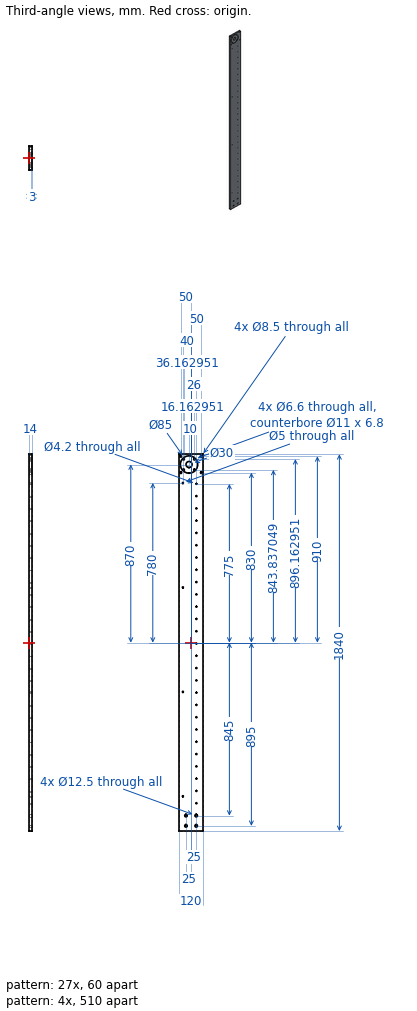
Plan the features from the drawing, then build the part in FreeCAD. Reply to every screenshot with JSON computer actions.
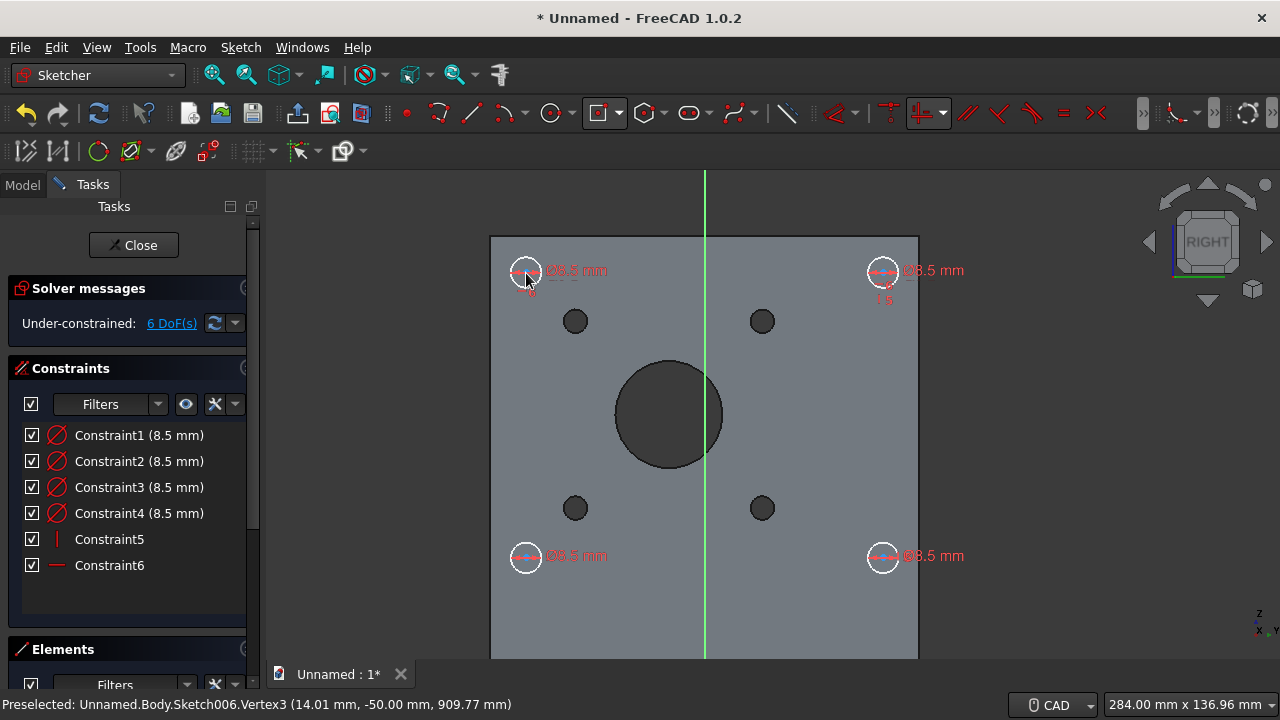
{"action": "left_click", "coordinate": [526, 273]}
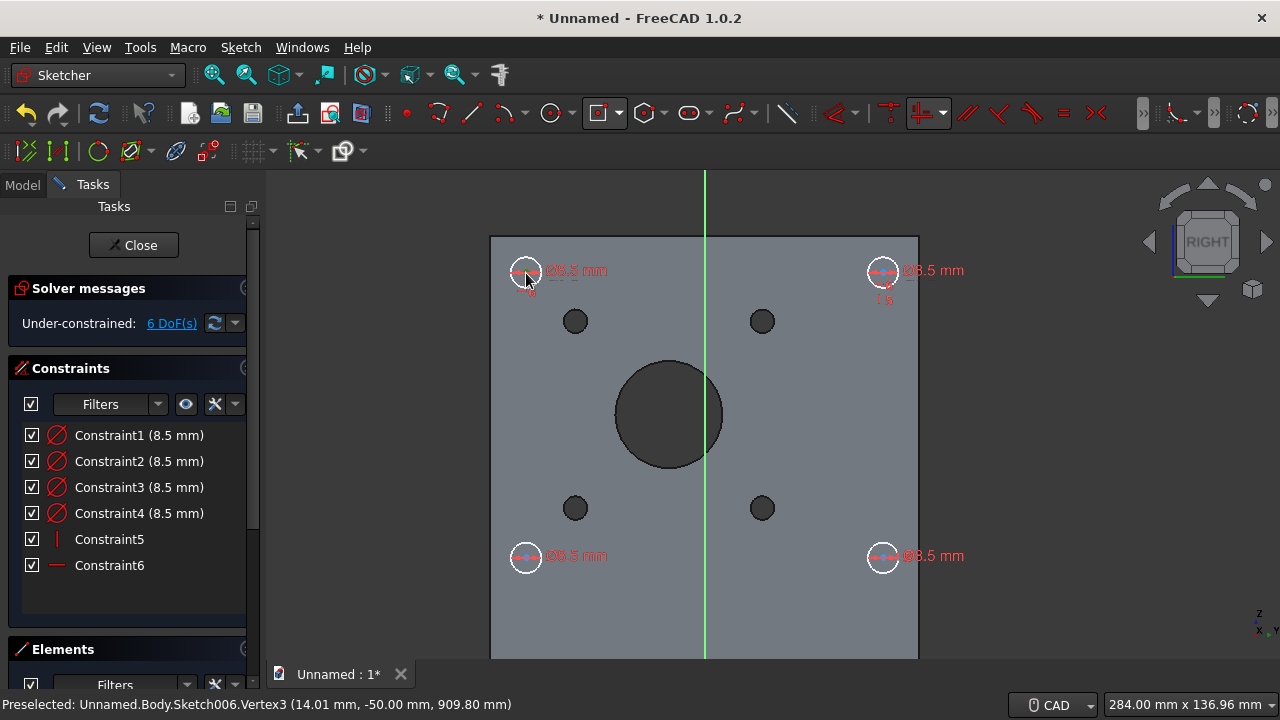
{"action": "left_click", "coordinate": [526, 558]}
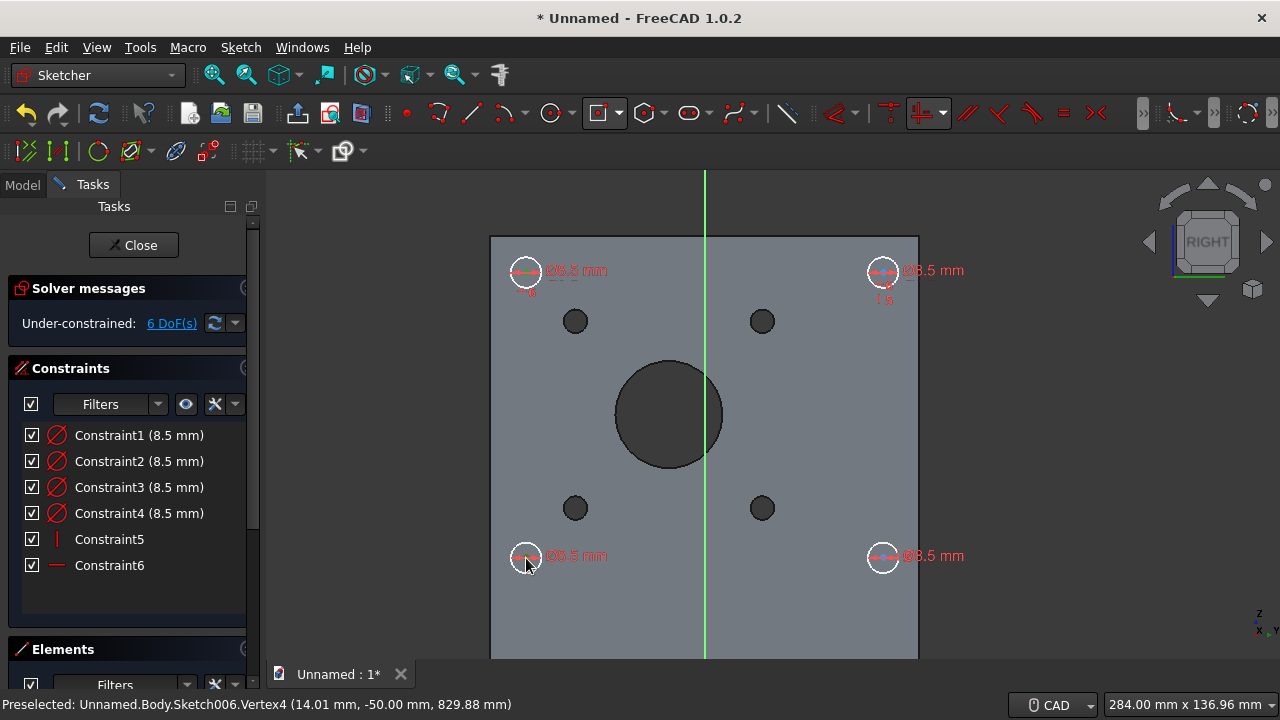
{"action": "key", "text": "v"}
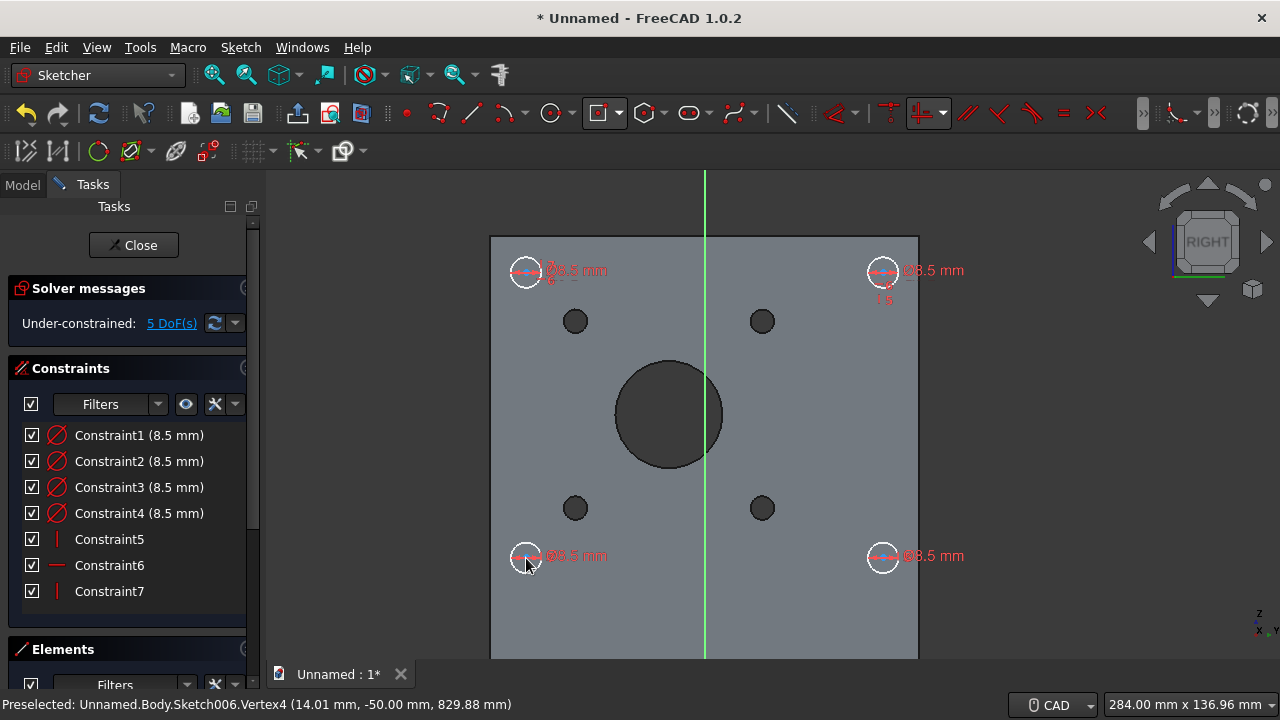
{"action": "left_click", "coordinate": [883, 558]}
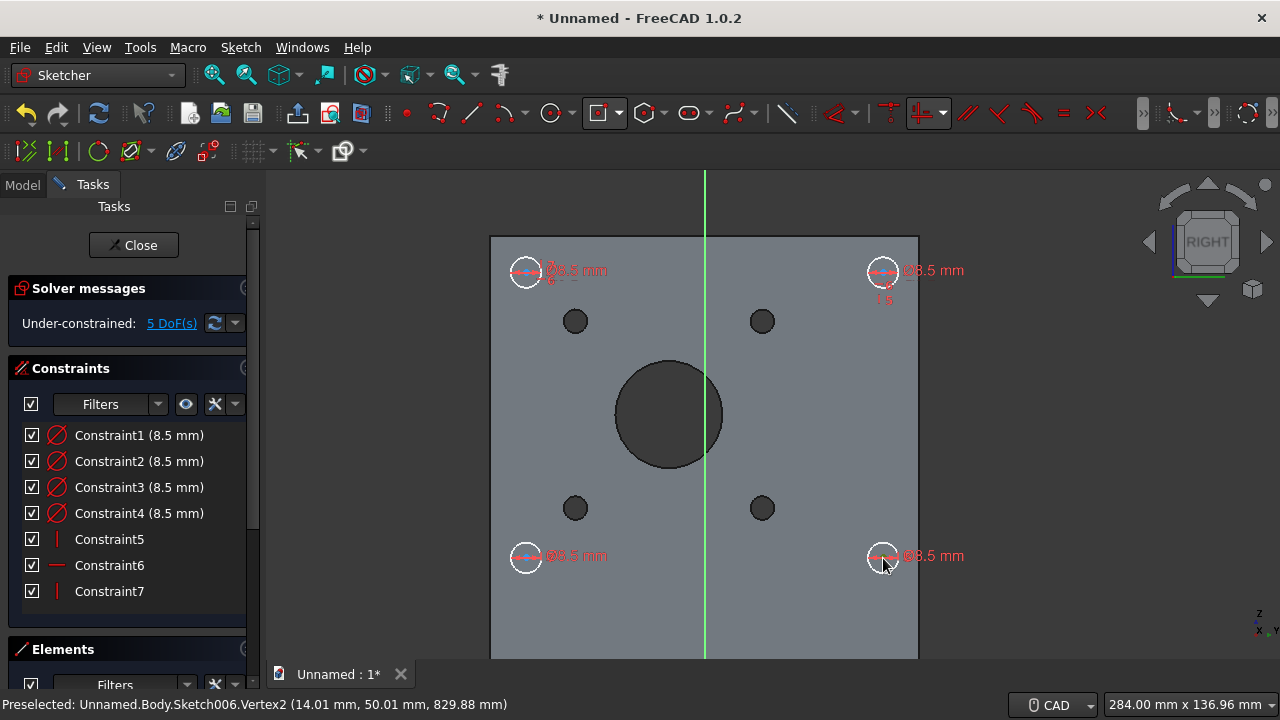
{"action": "left_click", "coordinate": [526, 558]}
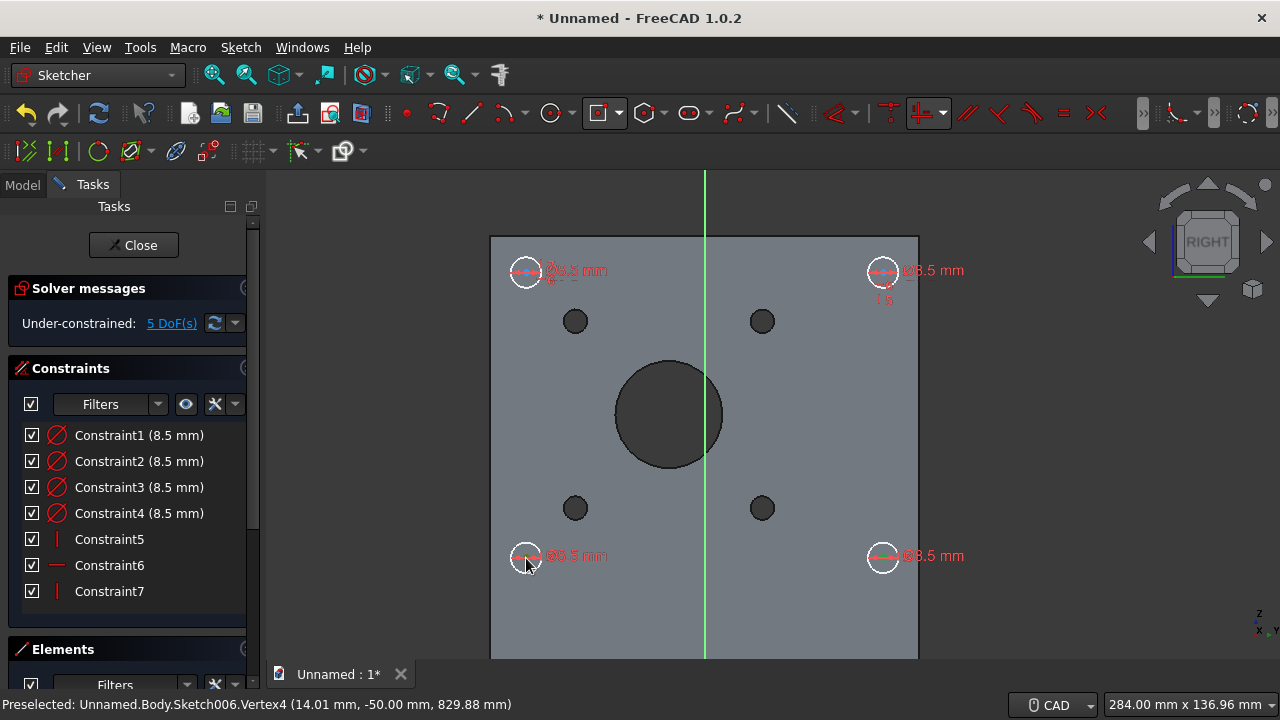
{"action": "key", "text": "h"}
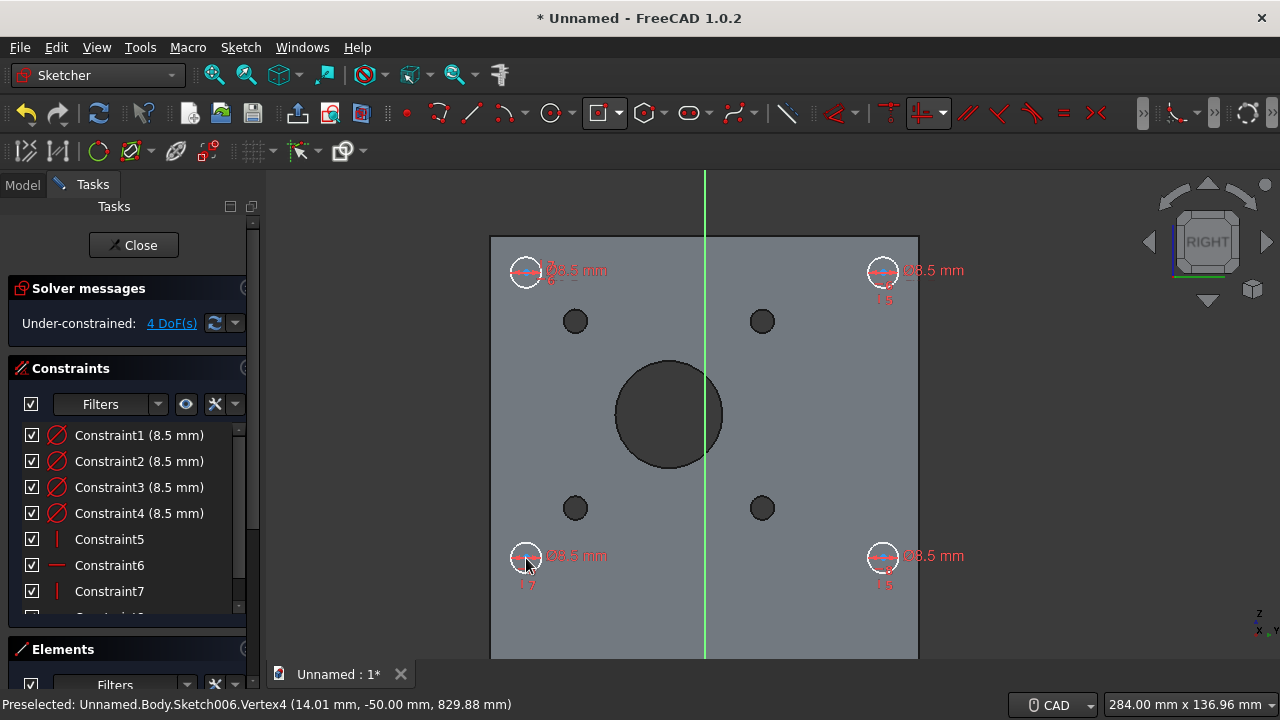
{"action": "left_click", "coordinate": [834, 114]}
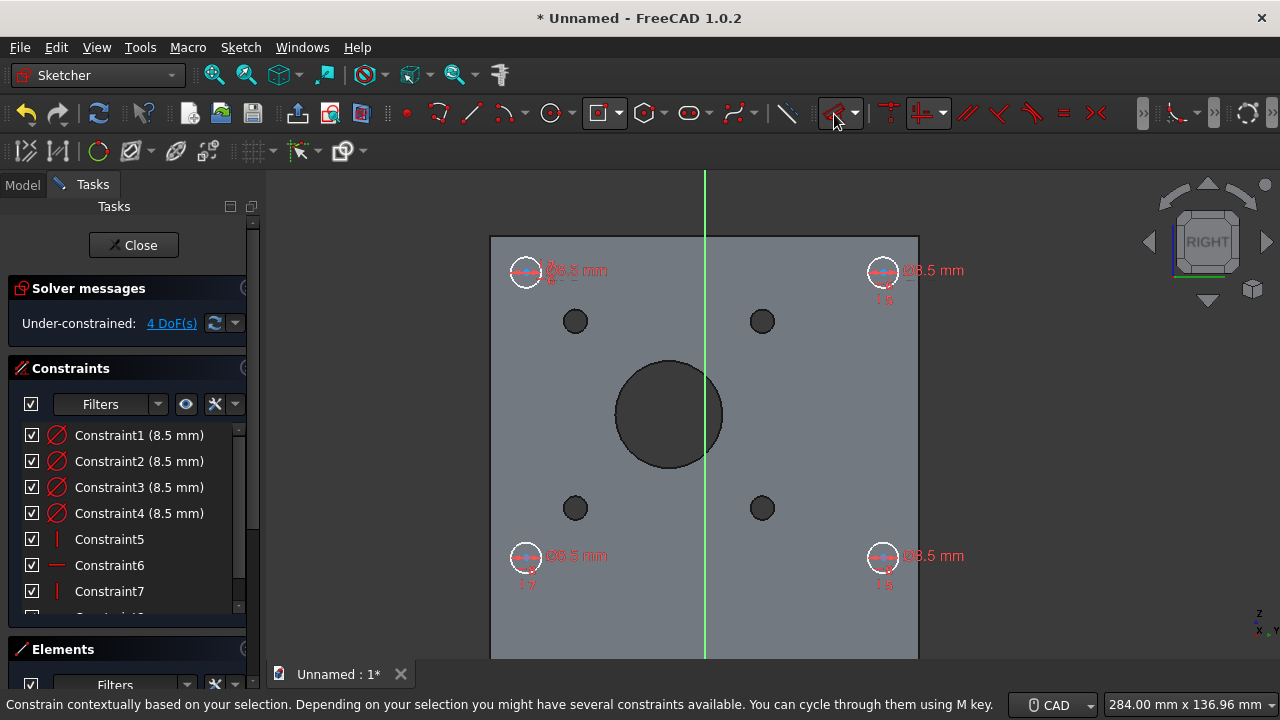
{"action": "left_click", "coordinate": [883, 273]}
{"action": "left_click", "coordinate": [794, 239]}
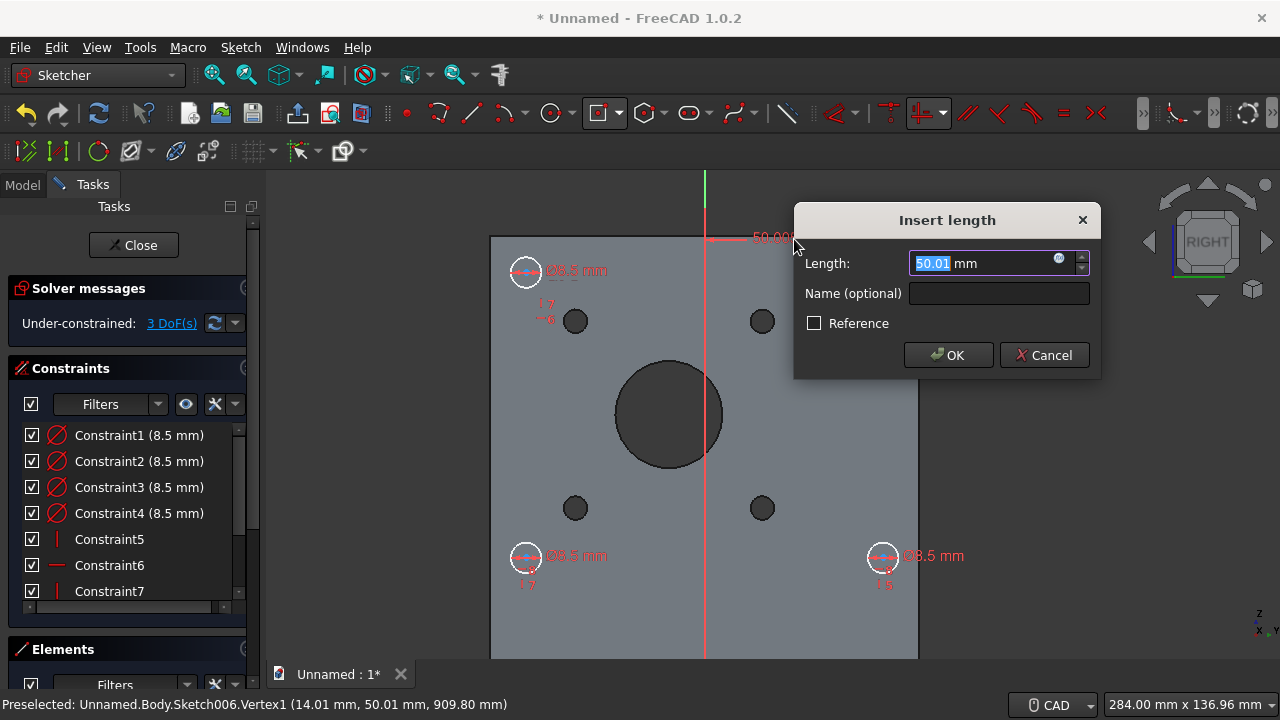
{"action": "type", "text": "50"}
{"action": "key", "text": "Return"}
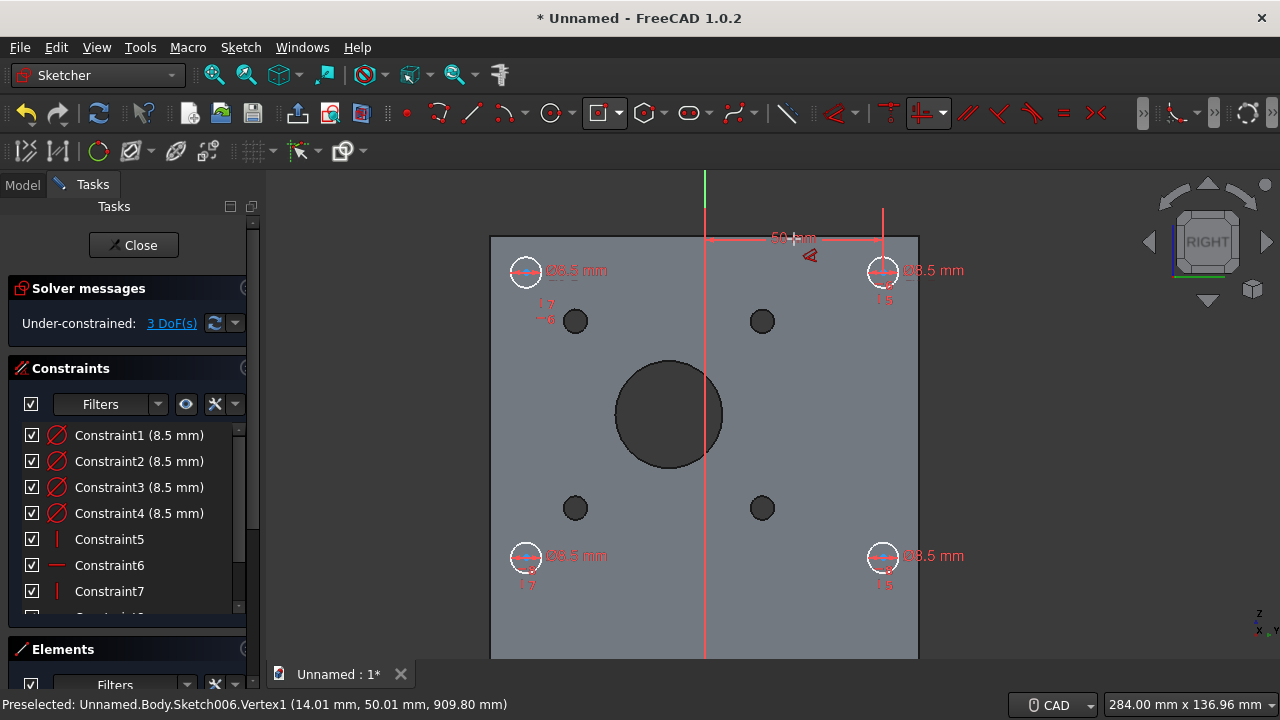
{"action": "left_click", "coordinate": [526, 273]}
{"action": "left_click", "coordinate": [615, 239]}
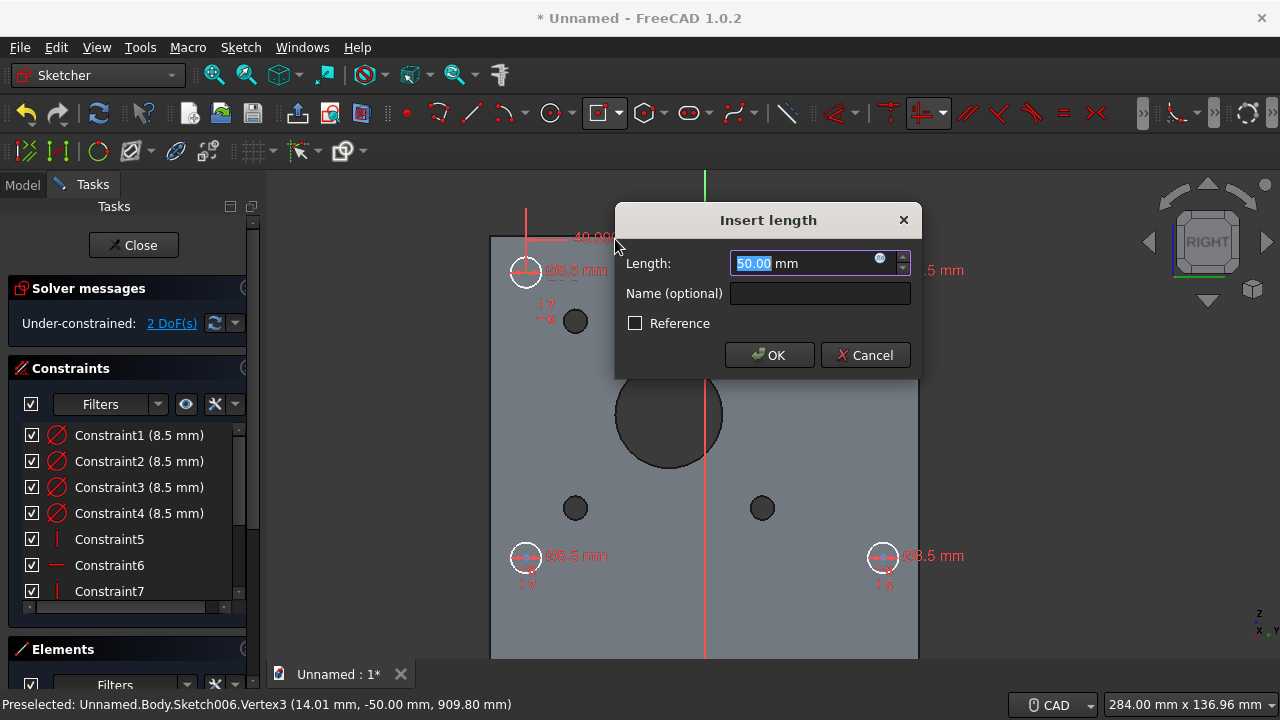
{"action": "type", "text": "50"}
{"action": "key", "text": "Return"}